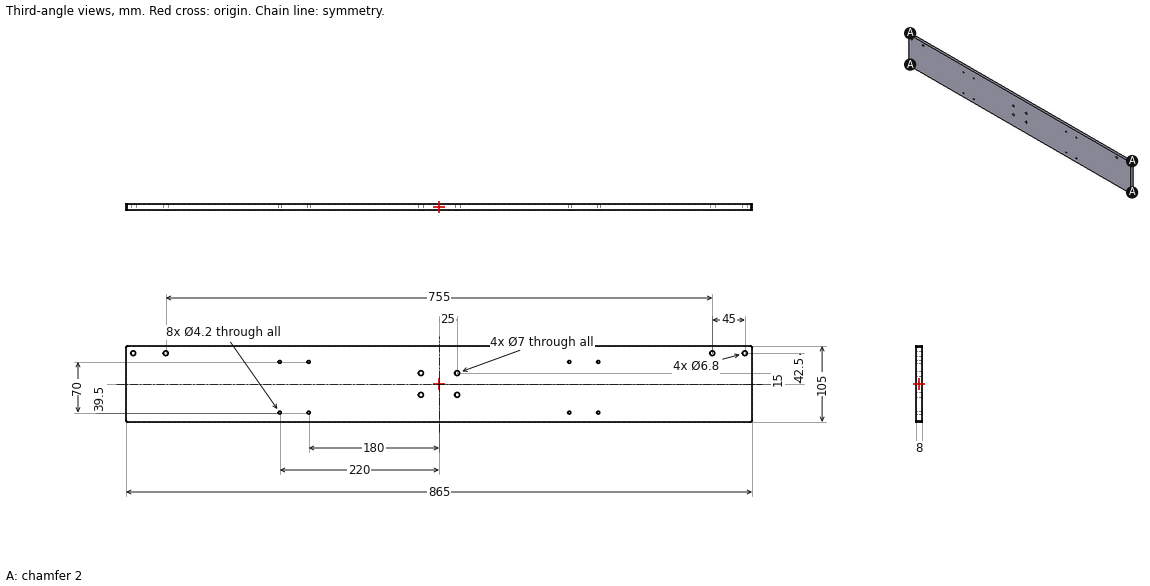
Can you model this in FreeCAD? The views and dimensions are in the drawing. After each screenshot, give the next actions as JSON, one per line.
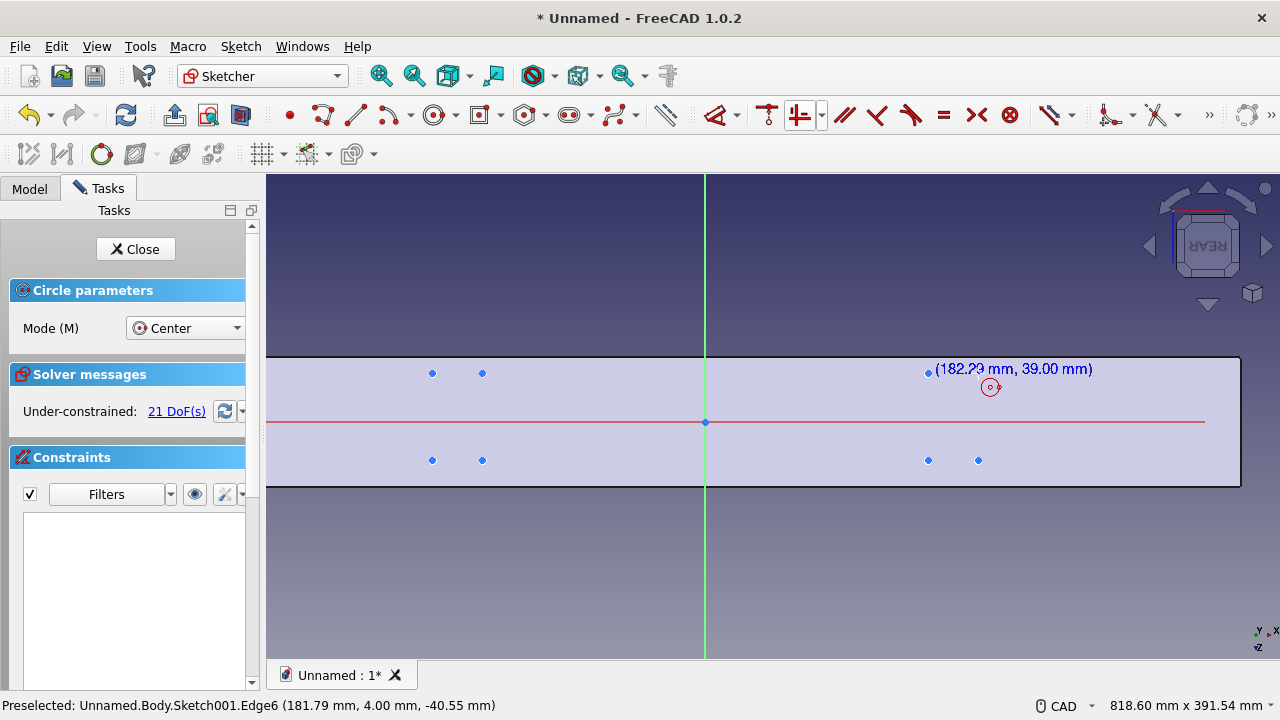
{"action": "left_click", "coordinate": [978, 373]}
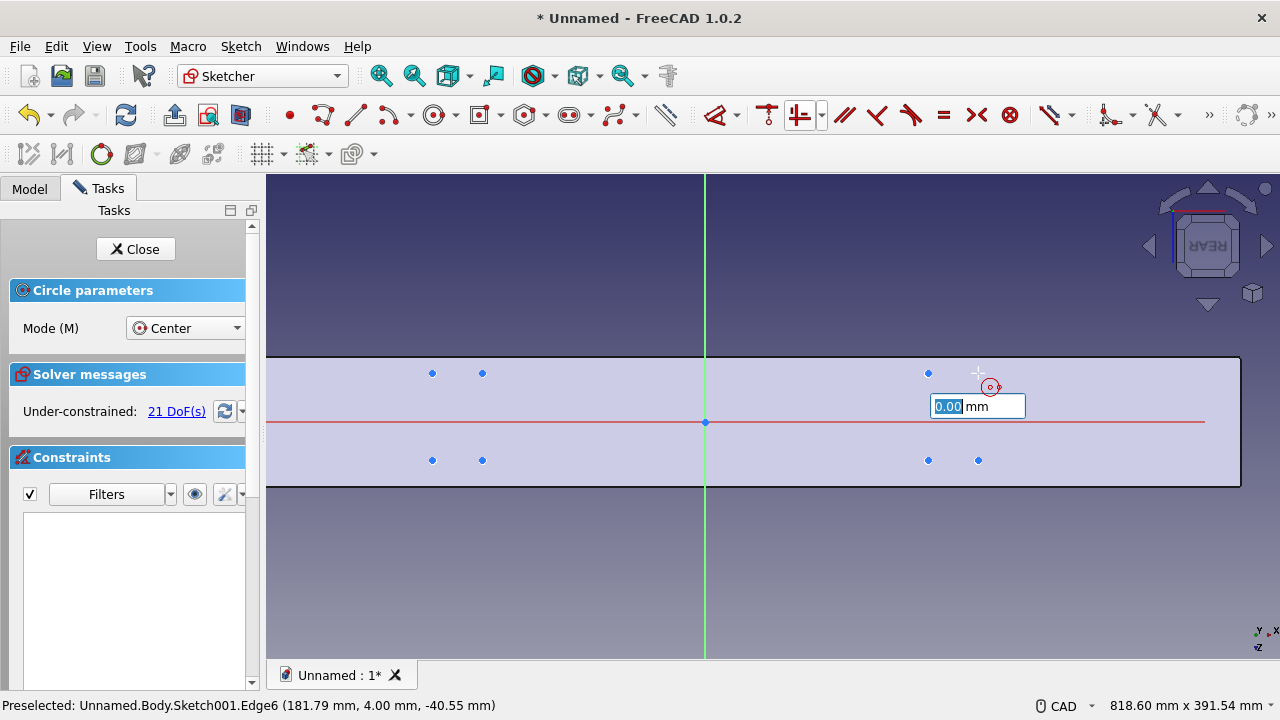
{"action": "scroll", "coordinate": [980, 372], "scroll_direction": "up", "scroll_amount": 10}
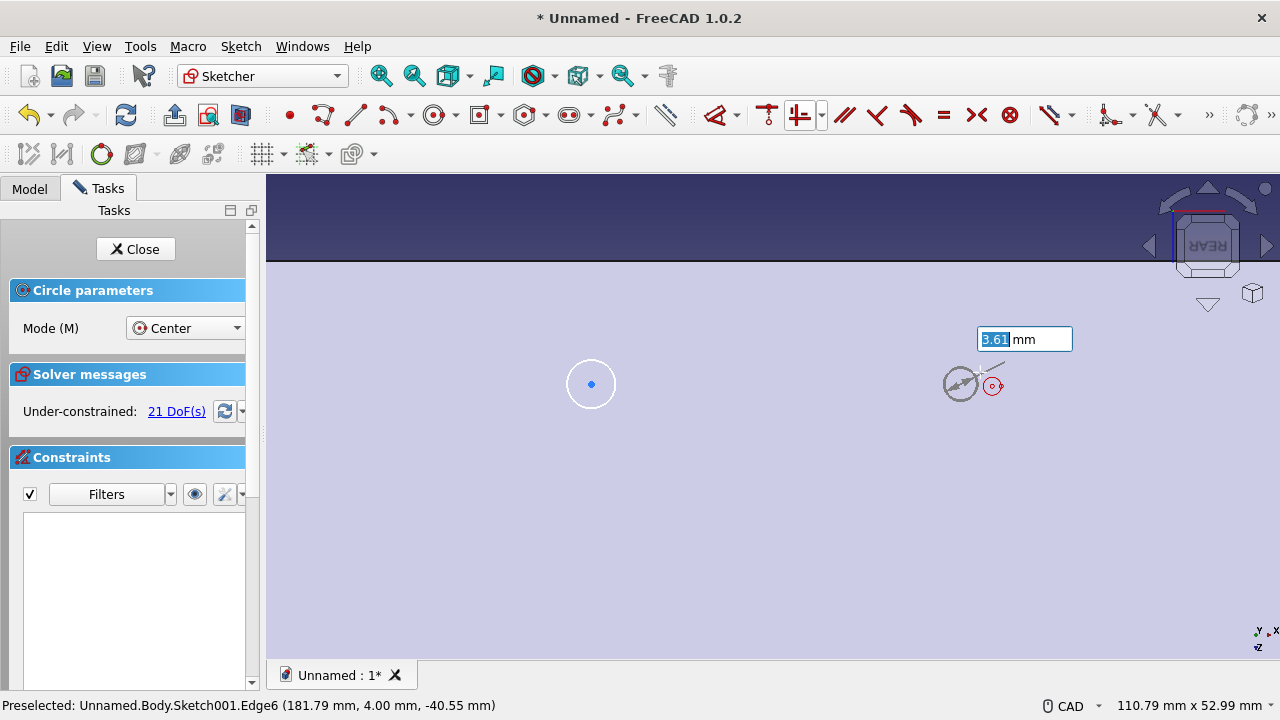
{"action": "left_click", "coordinate": [974, 366]}
{"action": "key", "text": "Escape"}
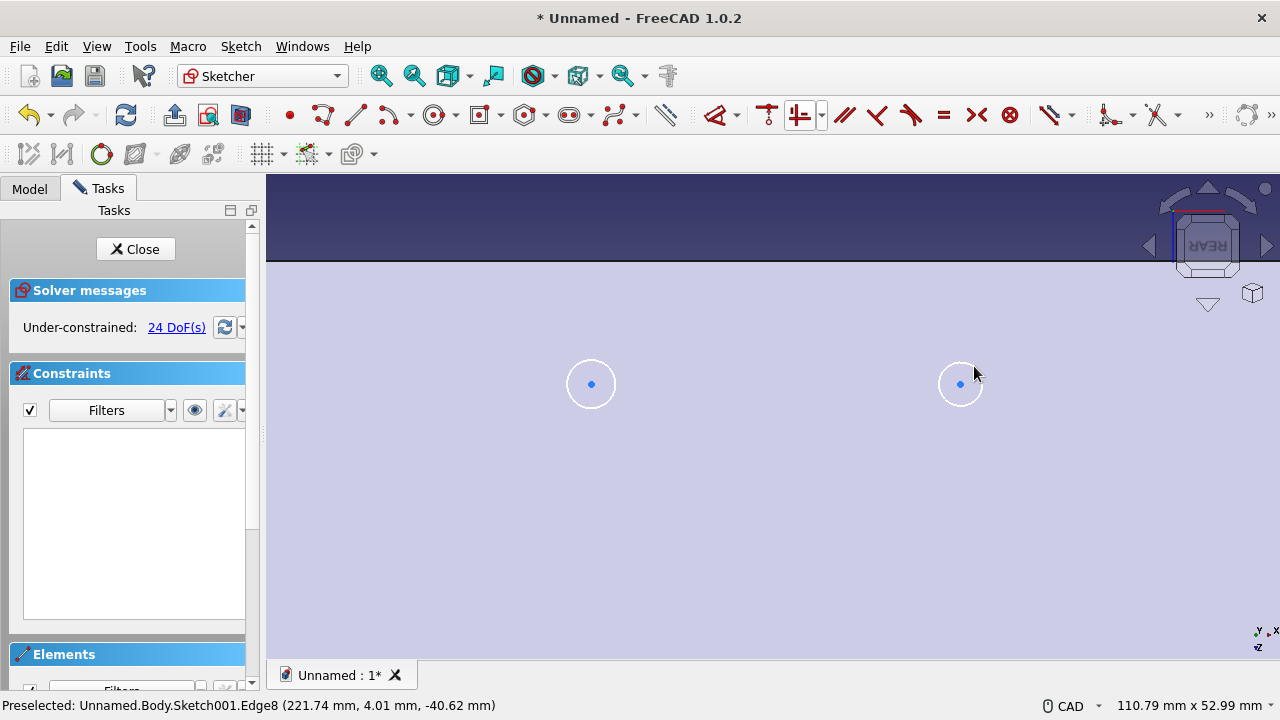
{"action": "scroll", "coordinate": [980, 372], "scroll_direction": "down", "scroll_amount": 10}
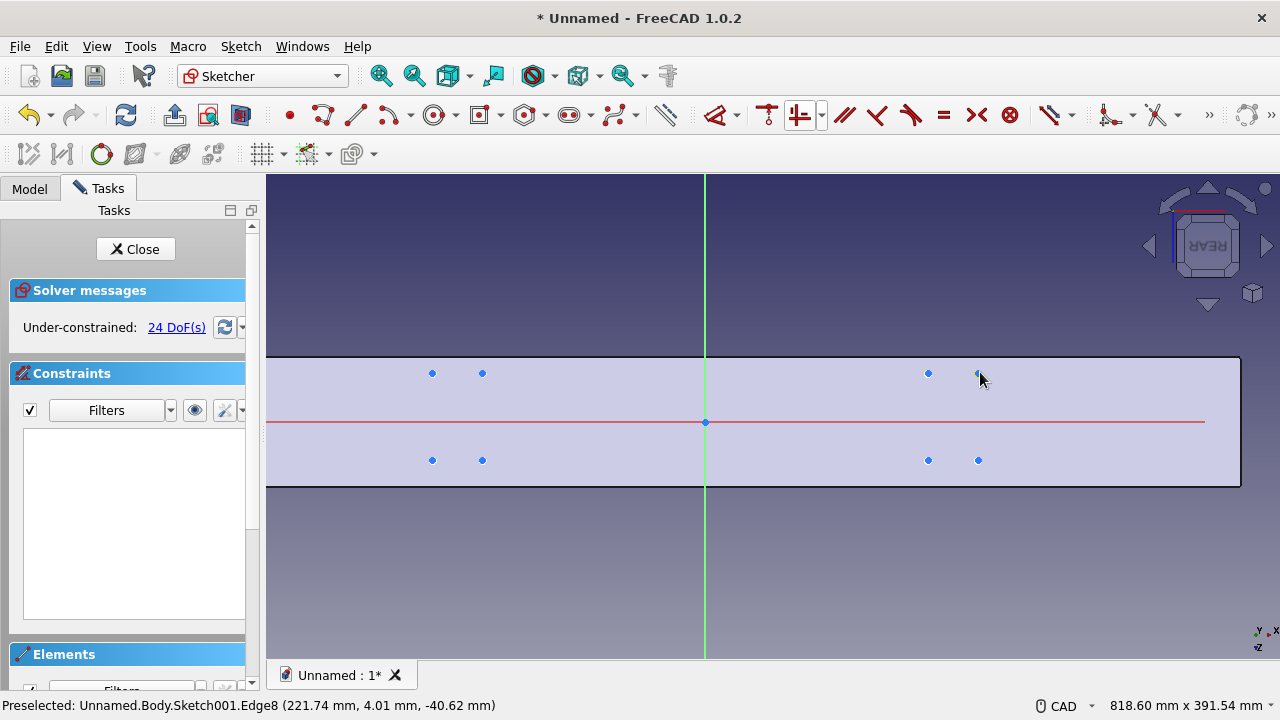
{"action": "scroll", "coordinate": [435, 372], "scroll_direction": "up", "scroll_amount": 8}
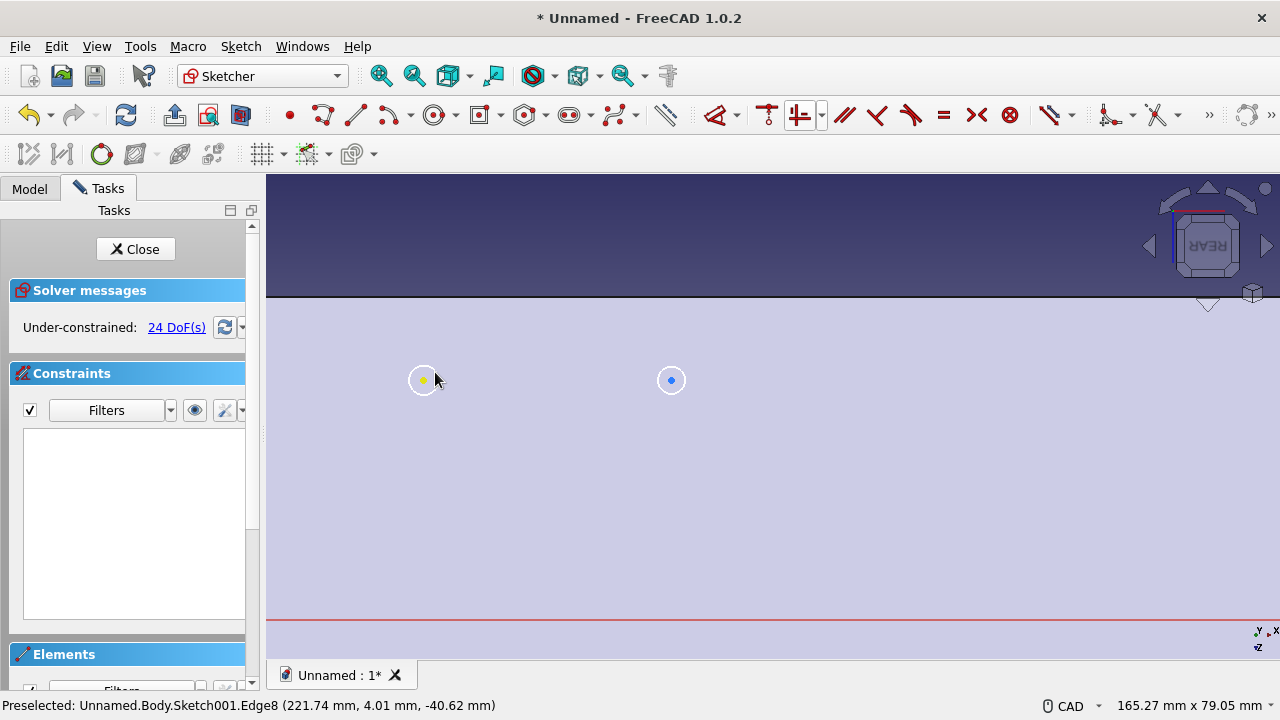
{"action": "left_click", "coordinate": [434, 370]}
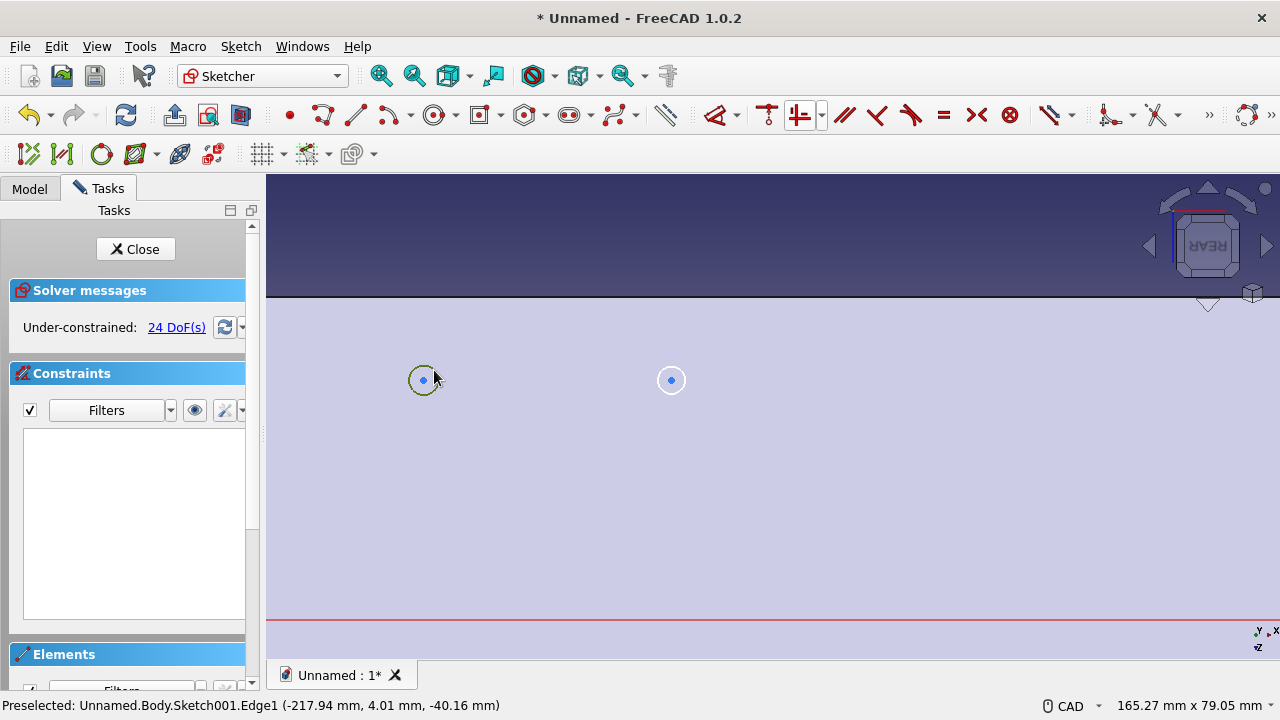
{"action": "left_click", "coordinate": [681, 371]}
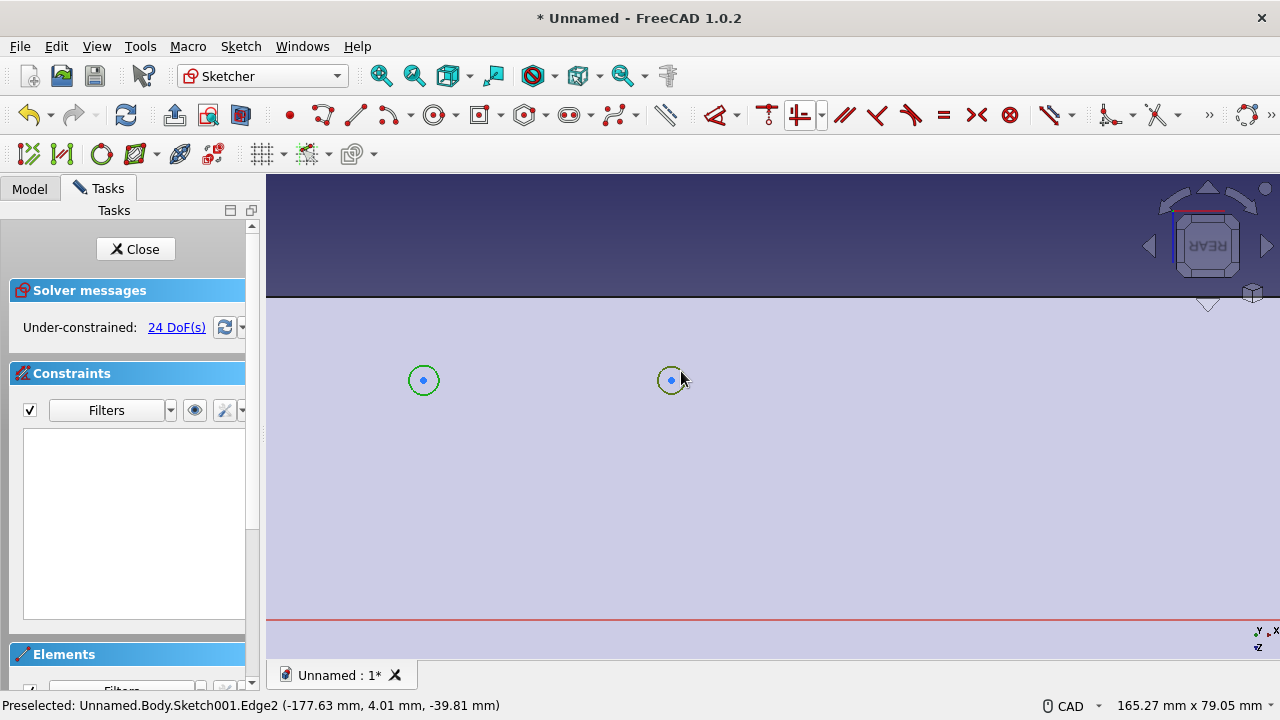
{"action": "scroll", "coordinate": [434, 372], "scroll_direction": "down", "scroll_amount": 8}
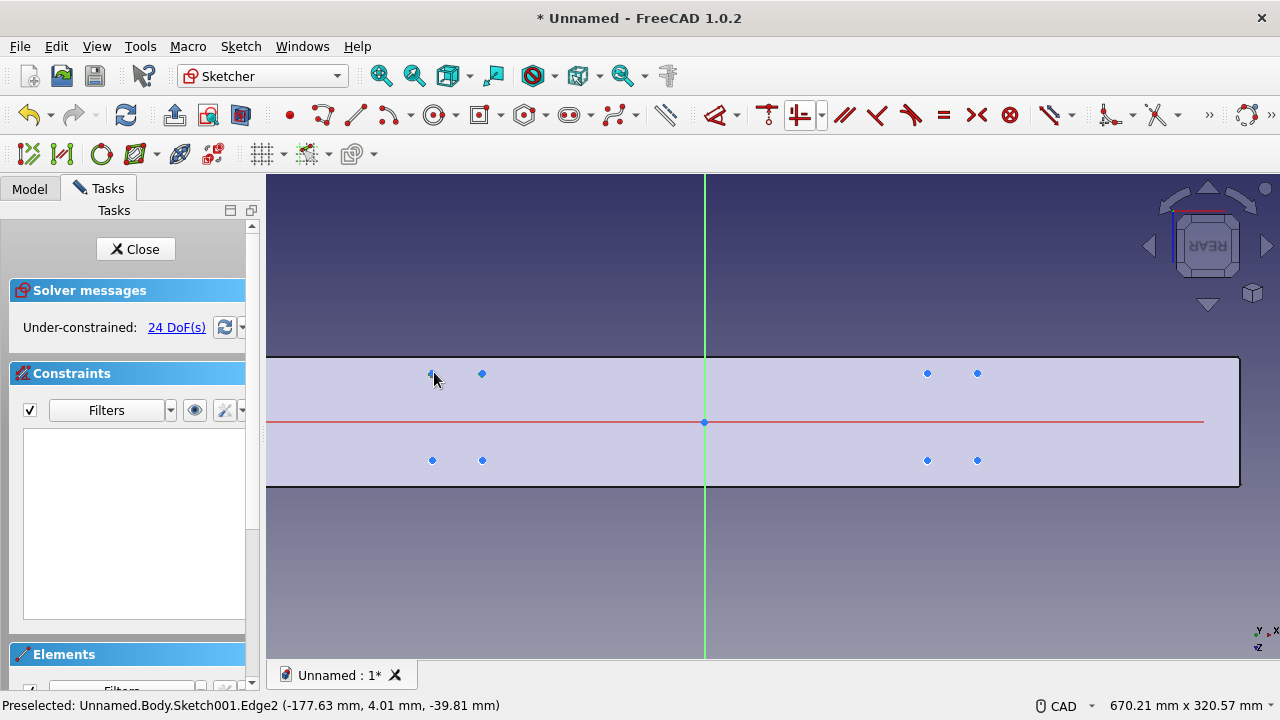
{"action": "scroll", "coordinate": [484, 459], "scroll_direction": "up", "scroll_amount": 8}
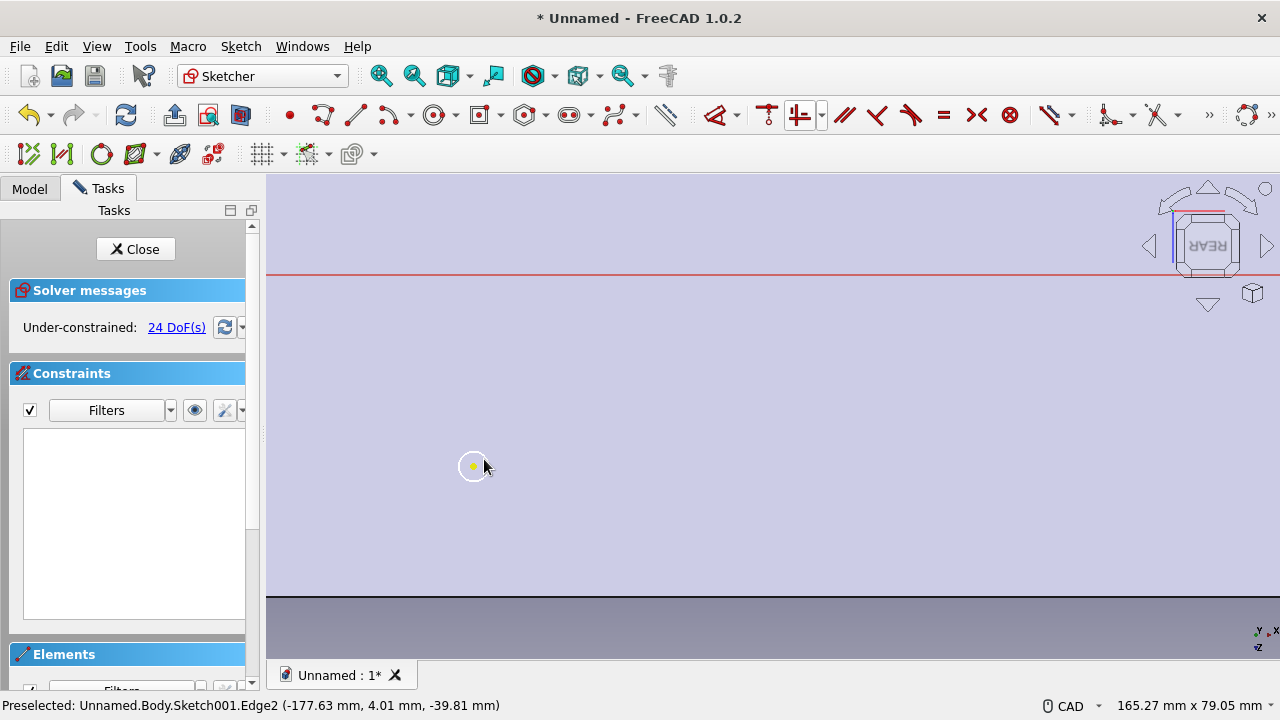
{"action": "left_click", "coordinate": [484, 456]}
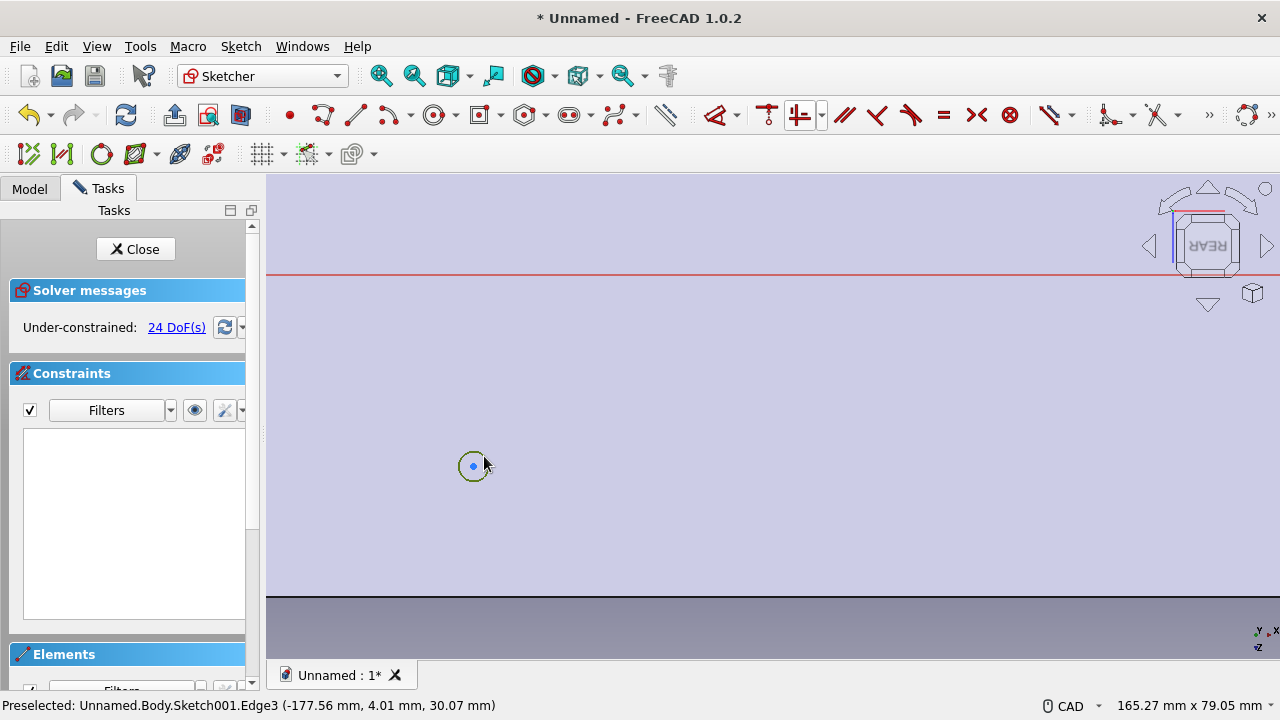
{"action": "scroll", "coordinate": [484, 459], "scroll_direction": "down", "scroll_amount": 8}